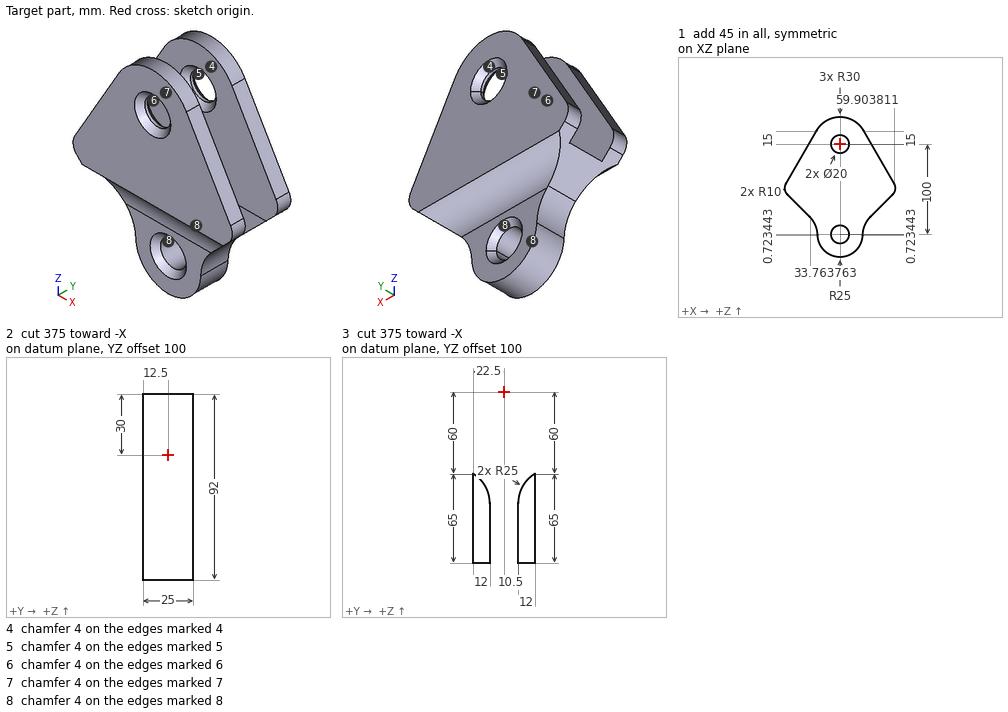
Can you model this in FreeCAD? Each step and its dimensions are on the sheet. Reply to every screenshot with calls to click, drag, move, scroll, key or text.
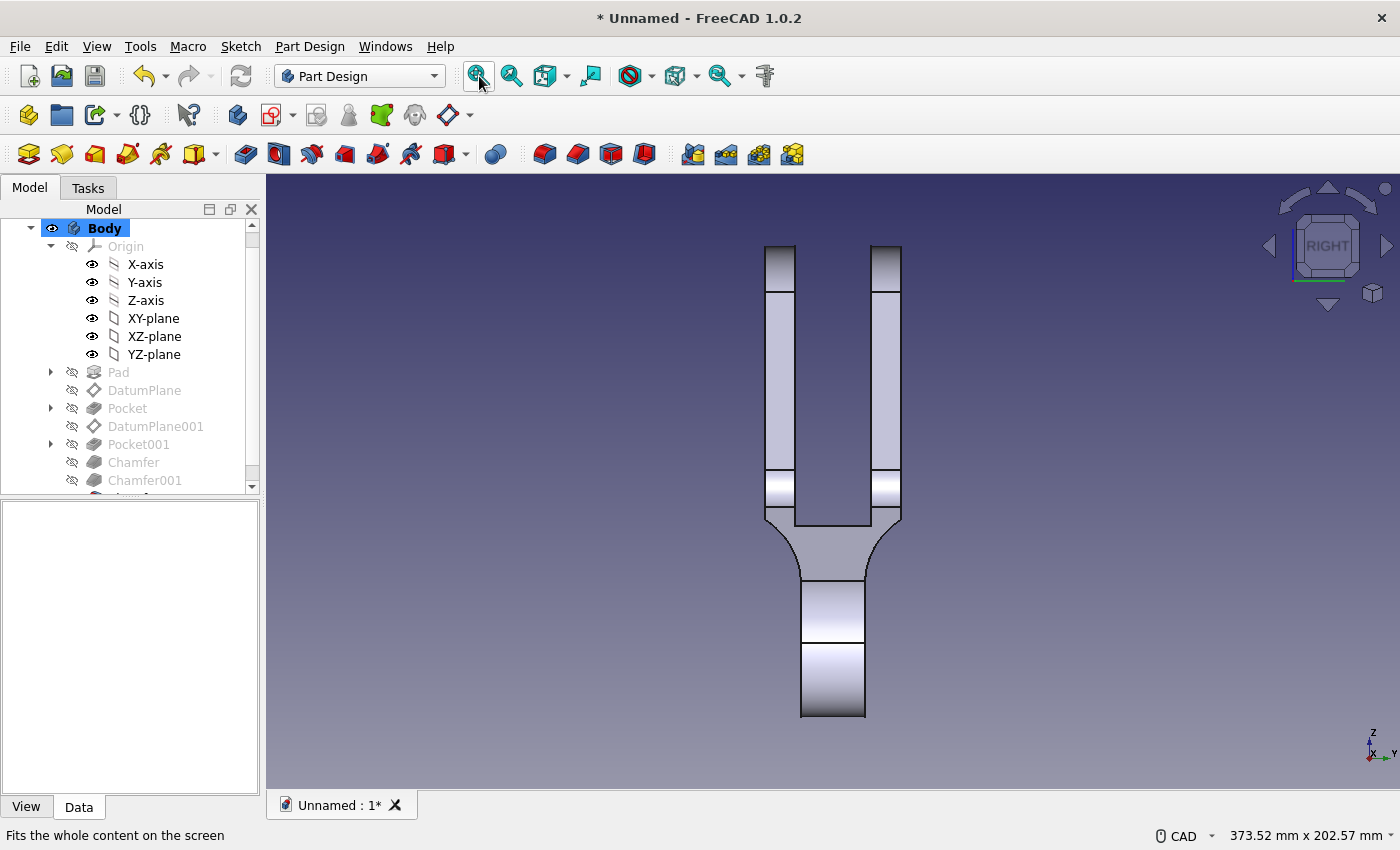
key(5)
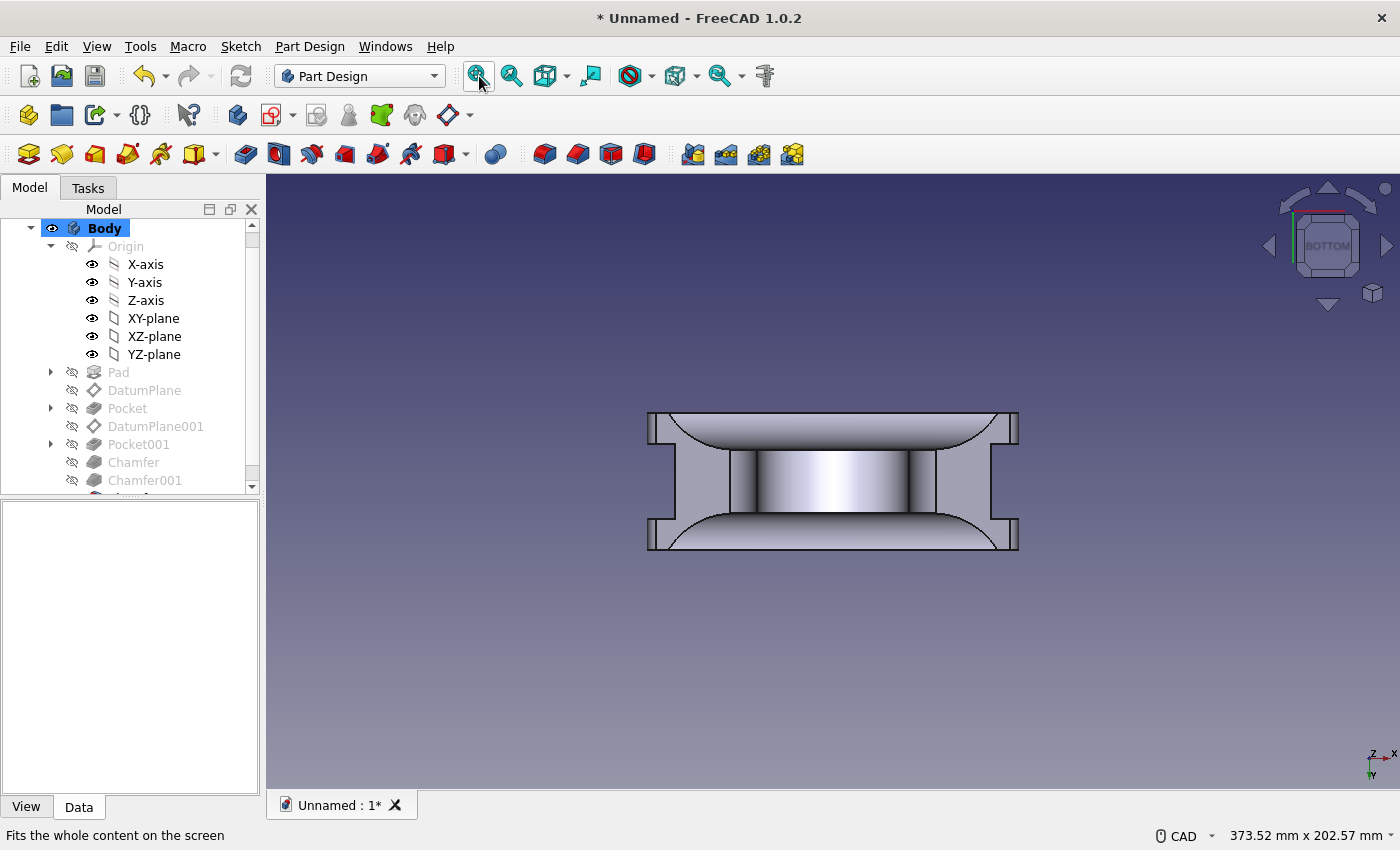
click(479, 76)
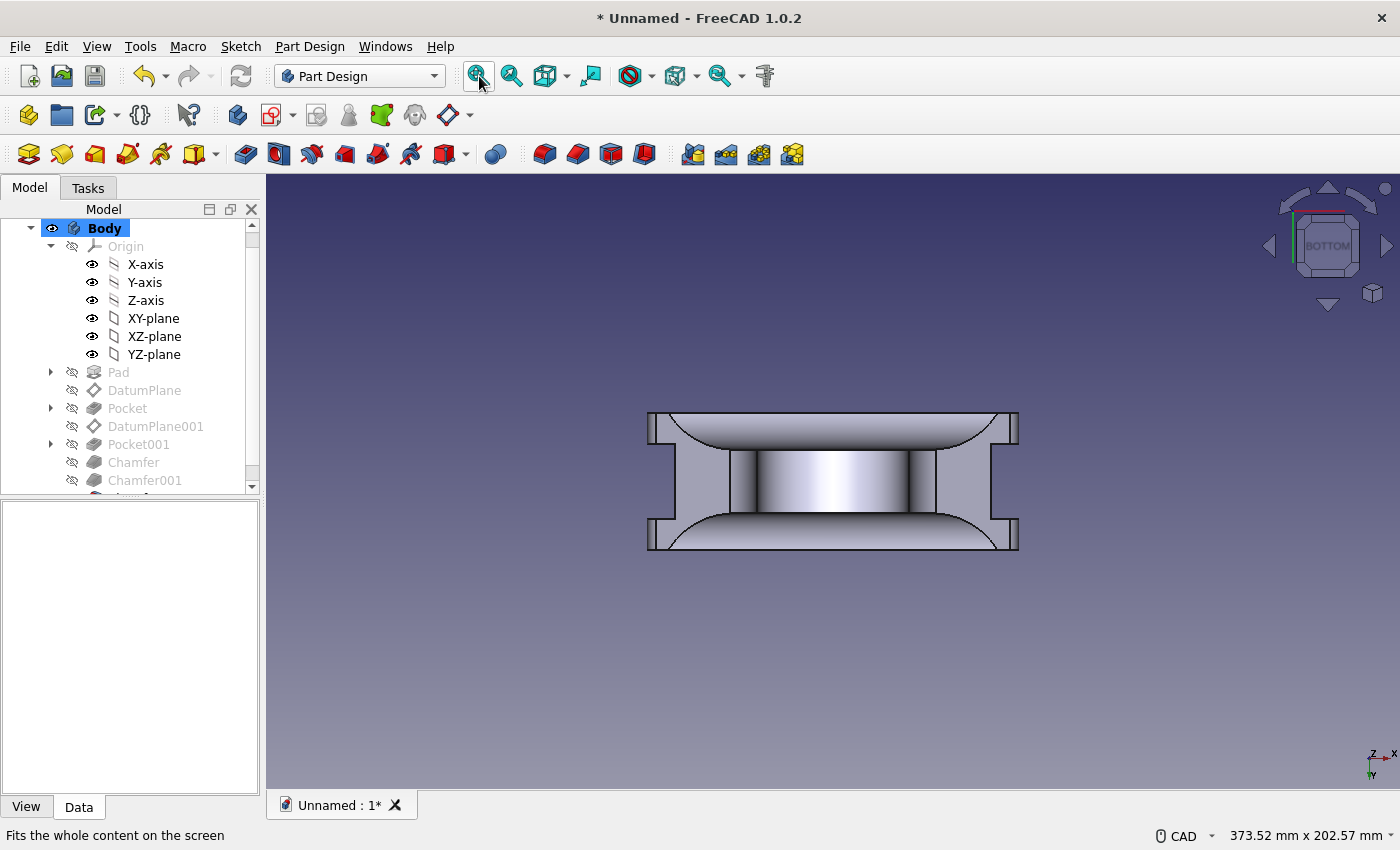
key(4)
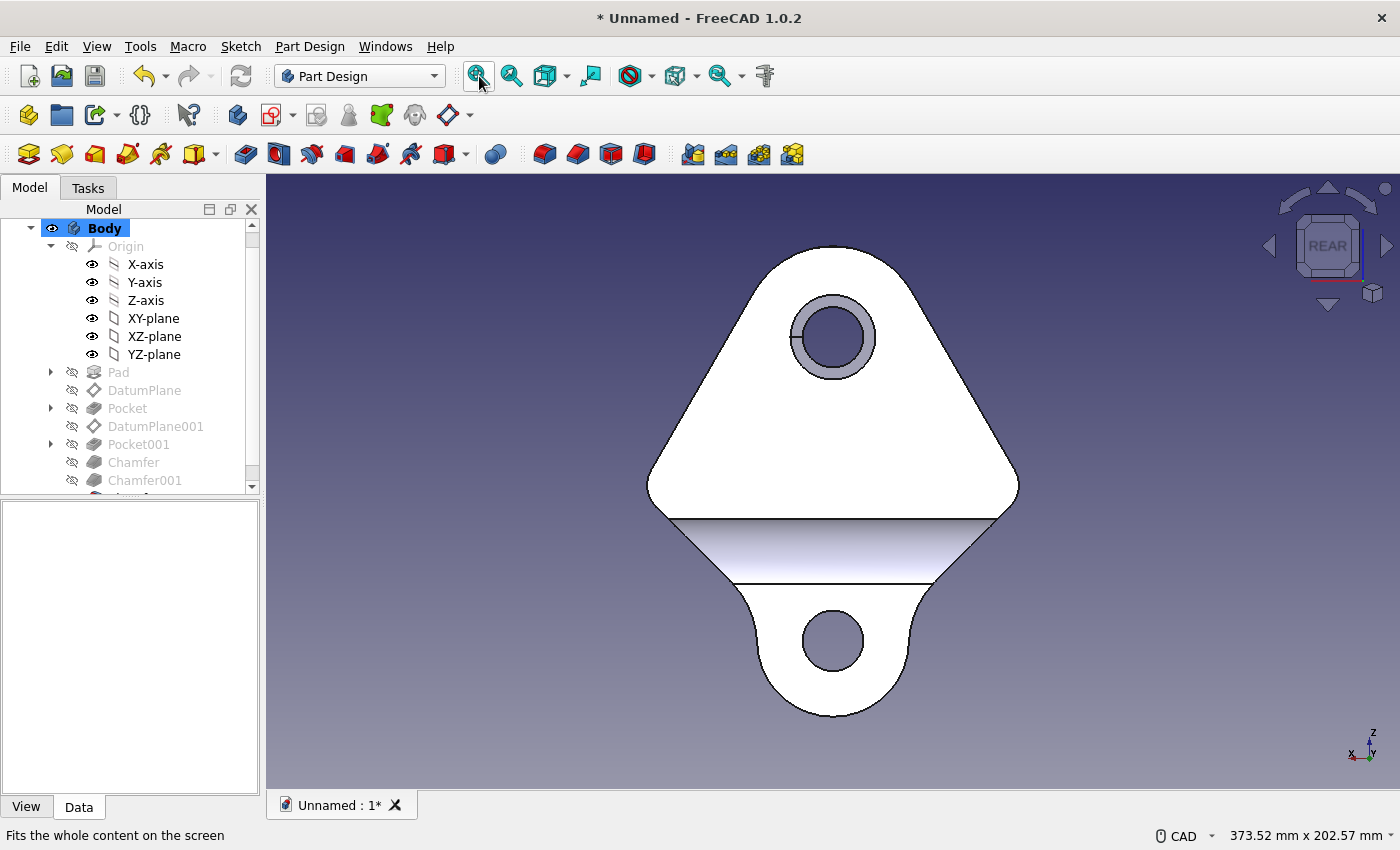
key(6)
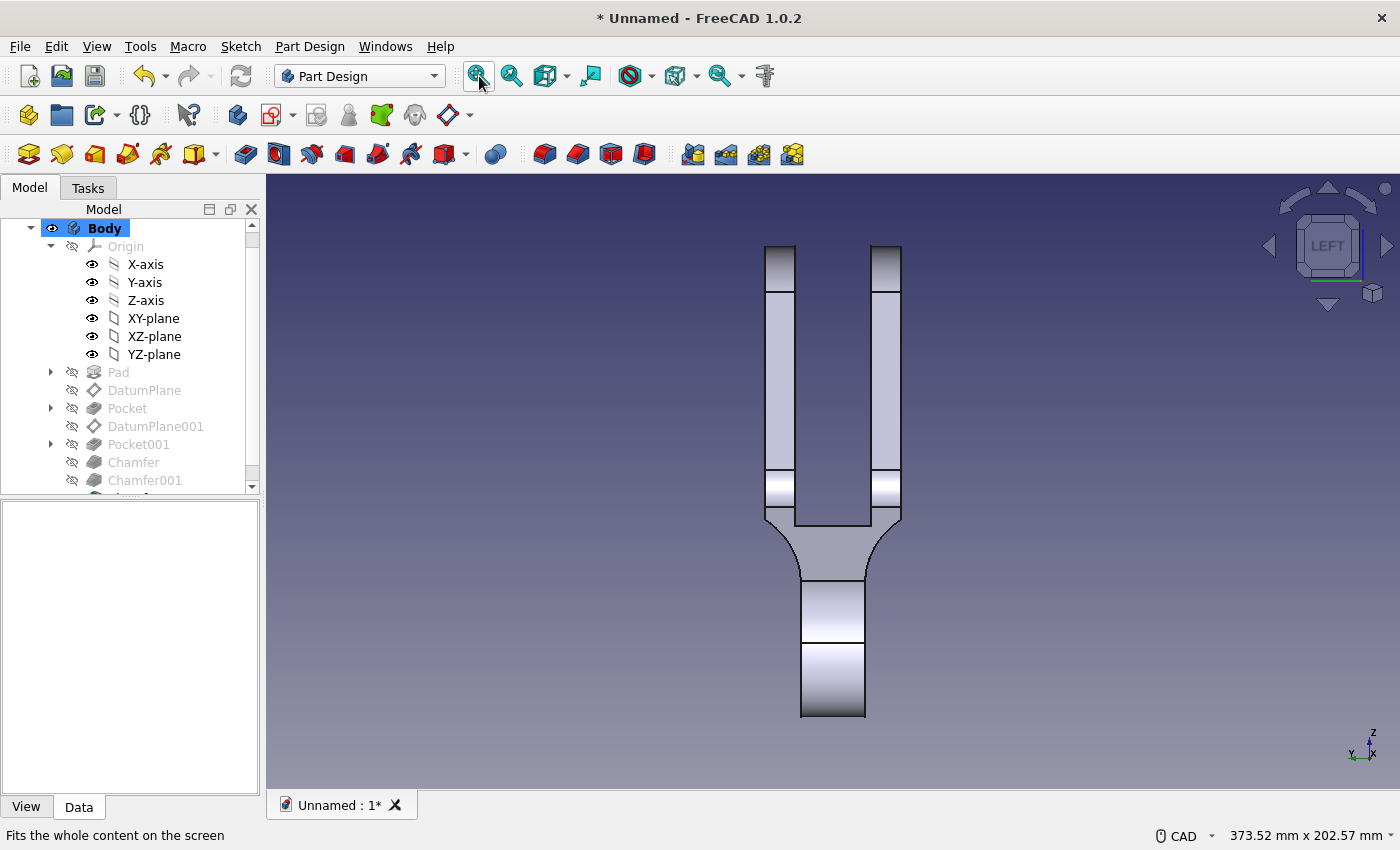
key(v)
key(3)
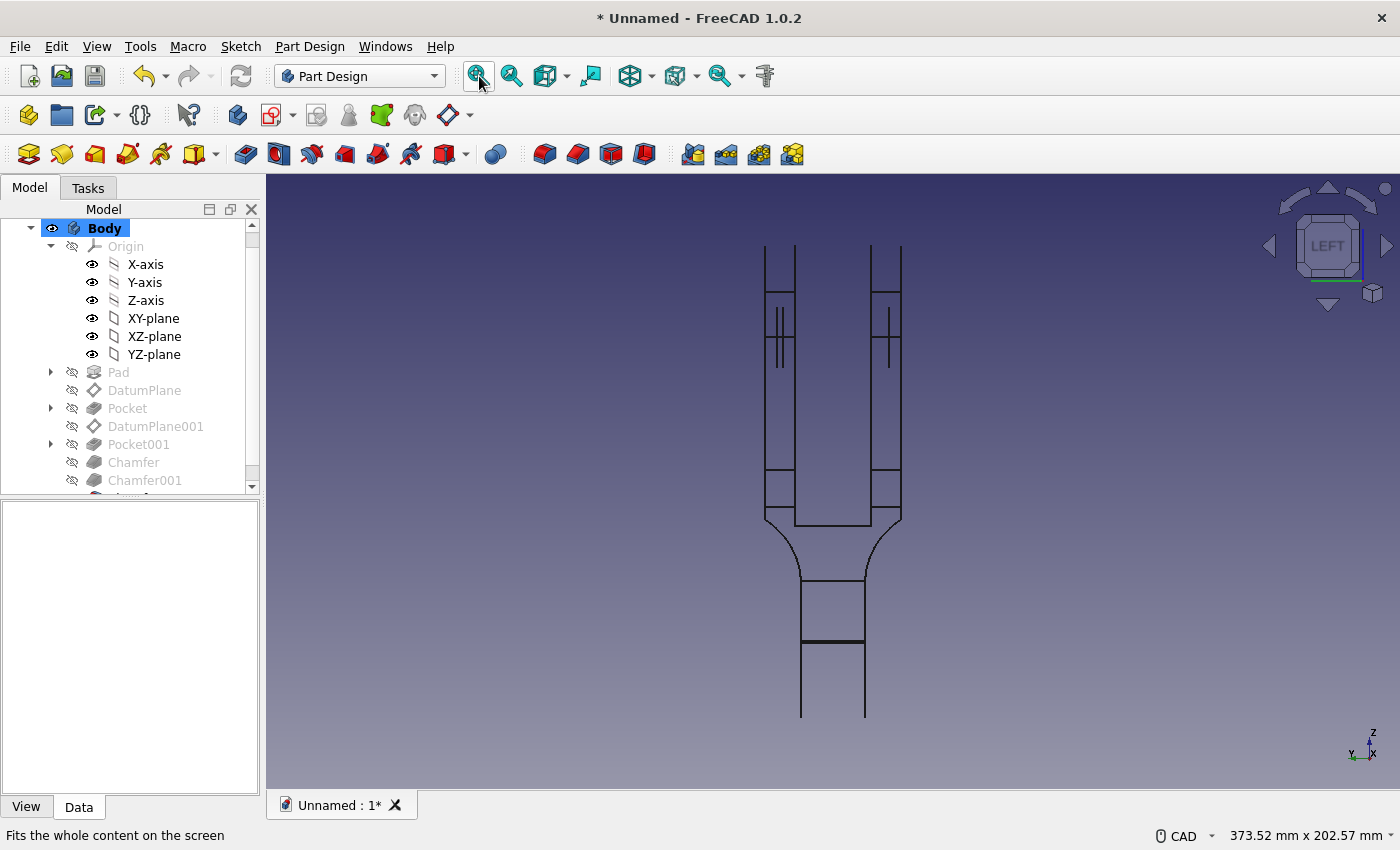
key(0)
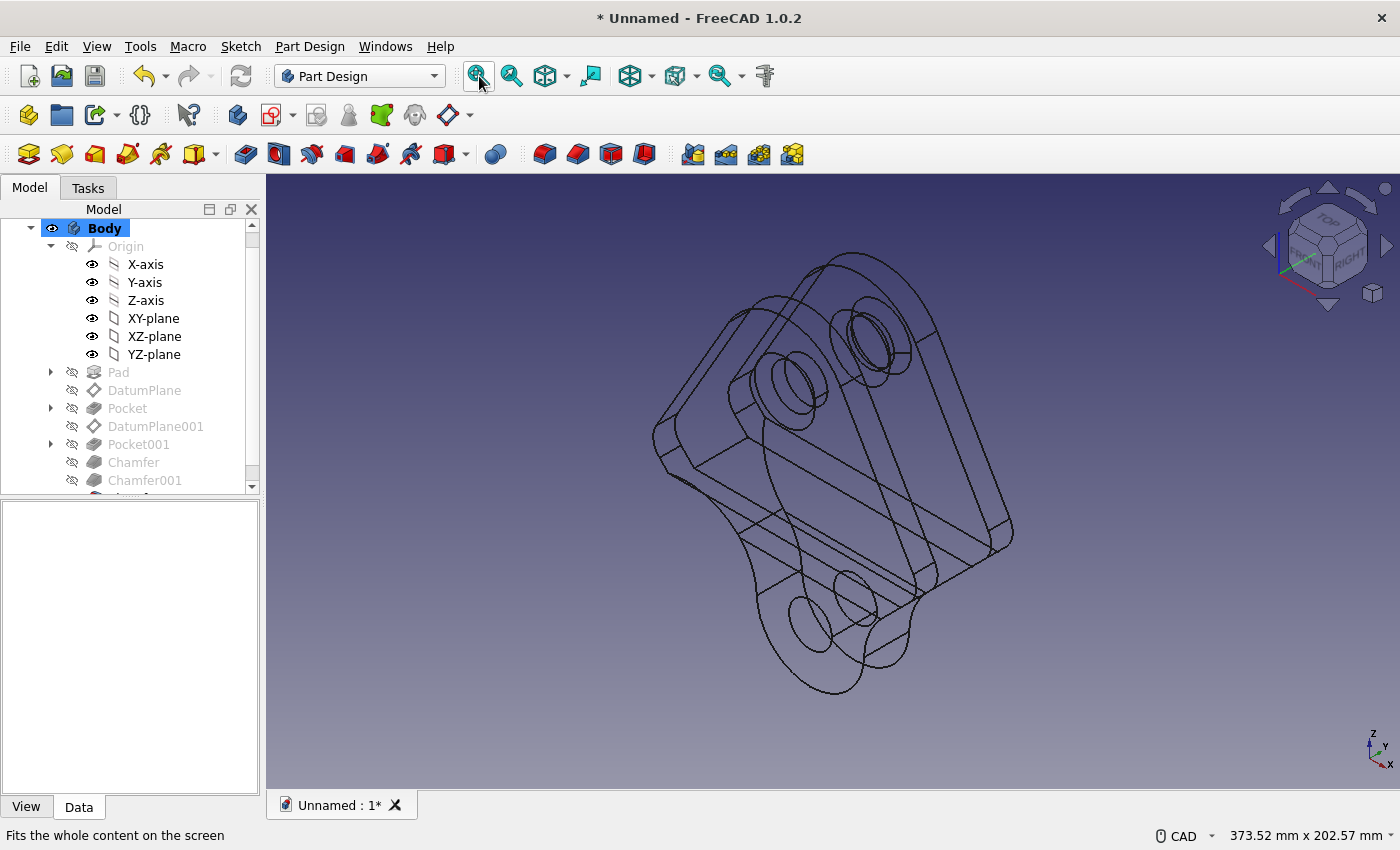
click(785, 366)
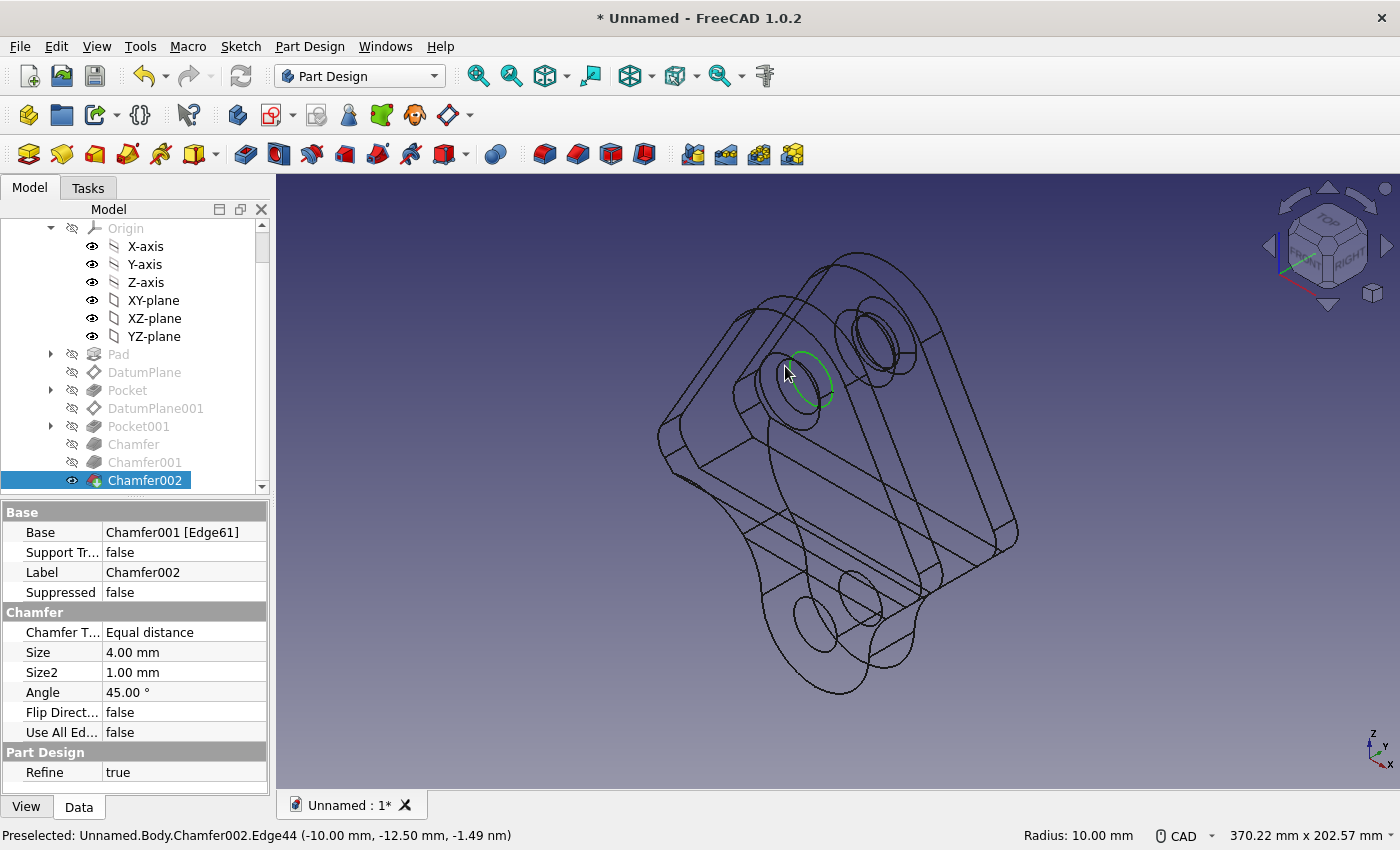
key(v)
key(1)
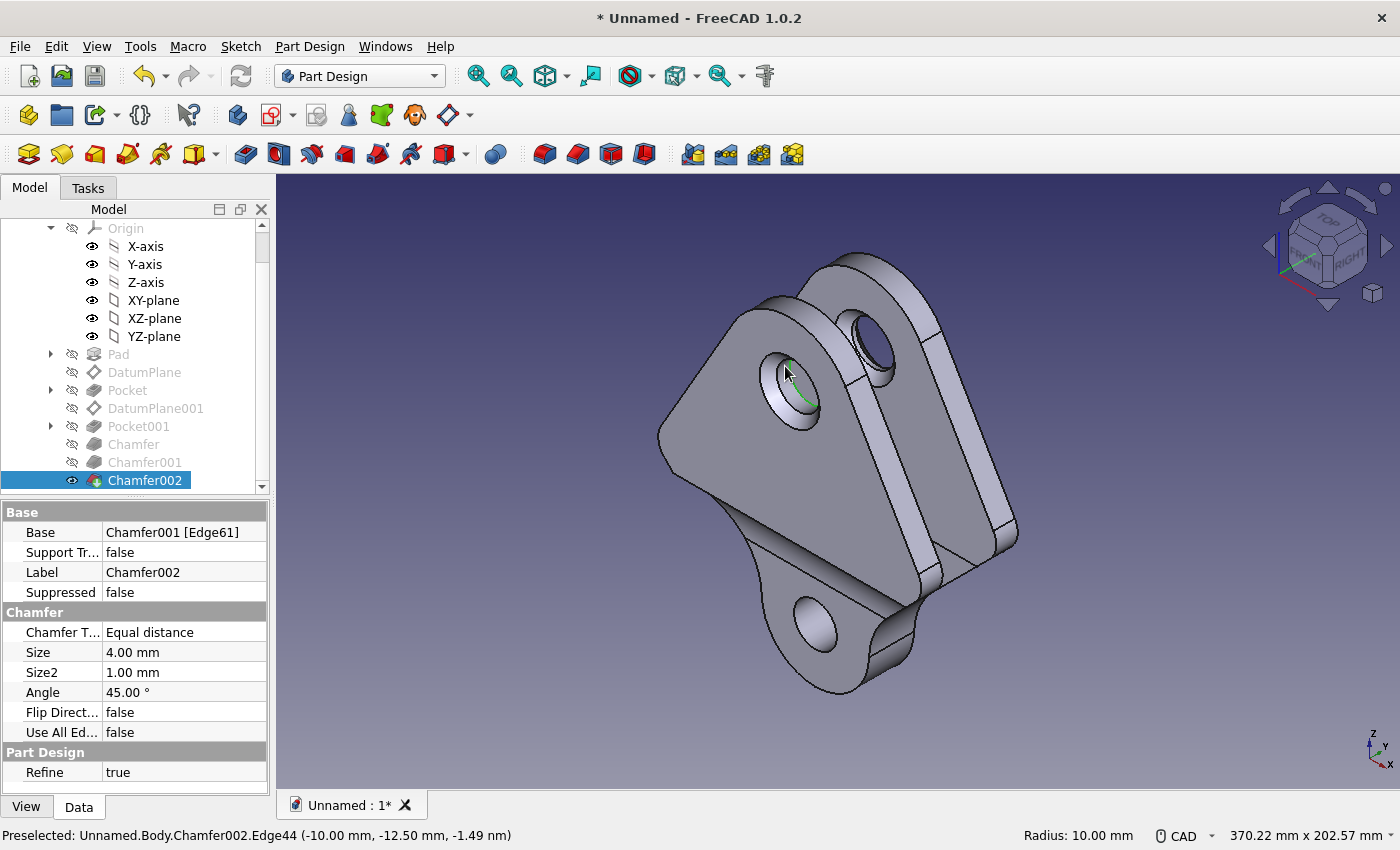
click(578, 154)